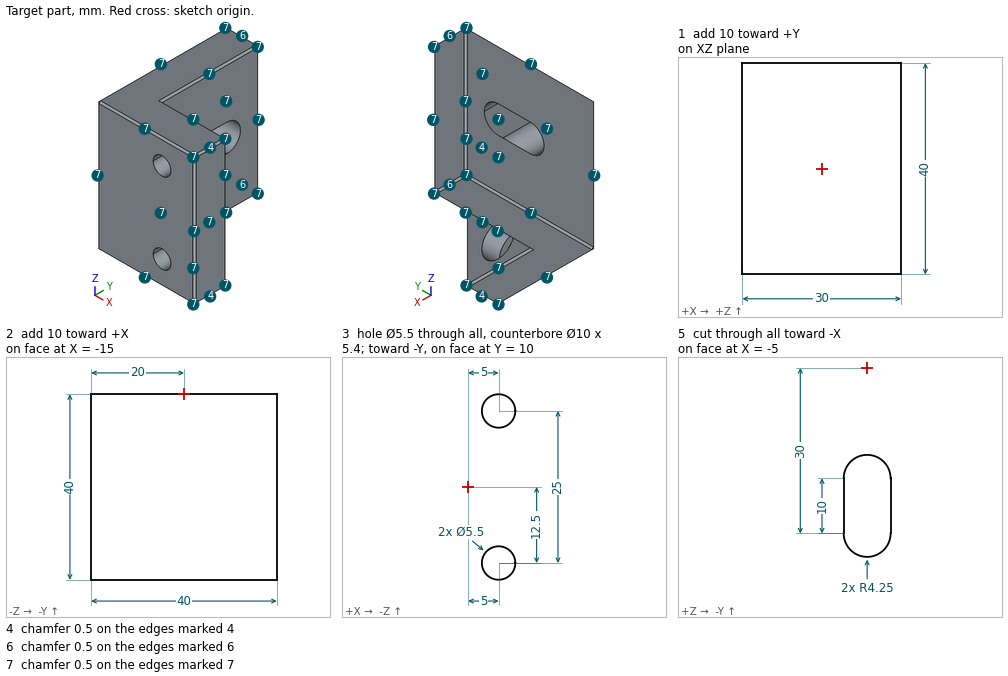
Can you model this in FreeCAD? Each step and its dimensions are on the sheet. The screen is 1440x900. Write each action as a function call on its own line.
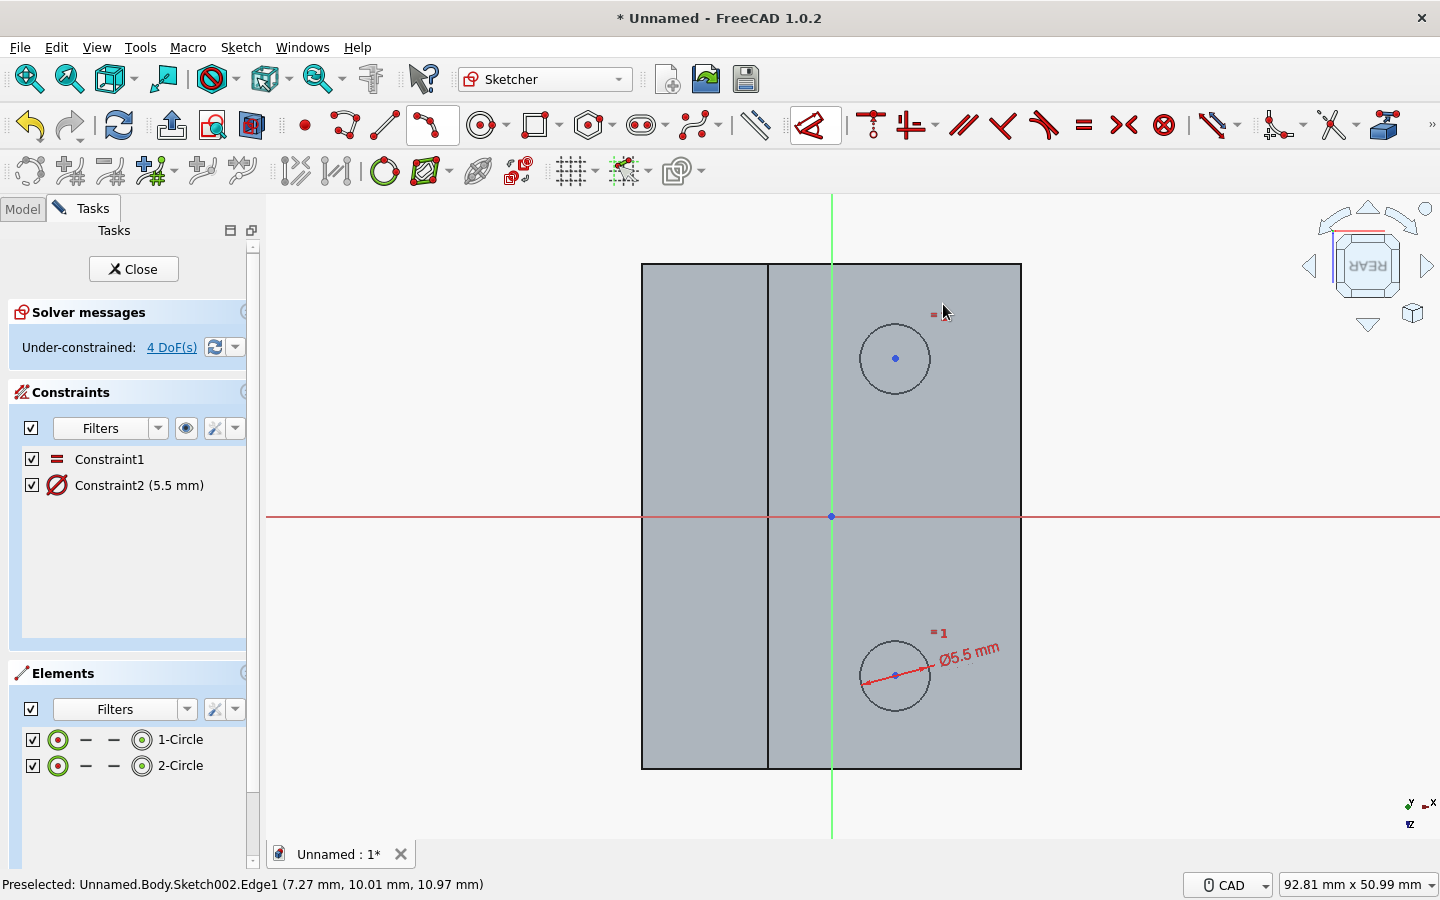
click(895, 676)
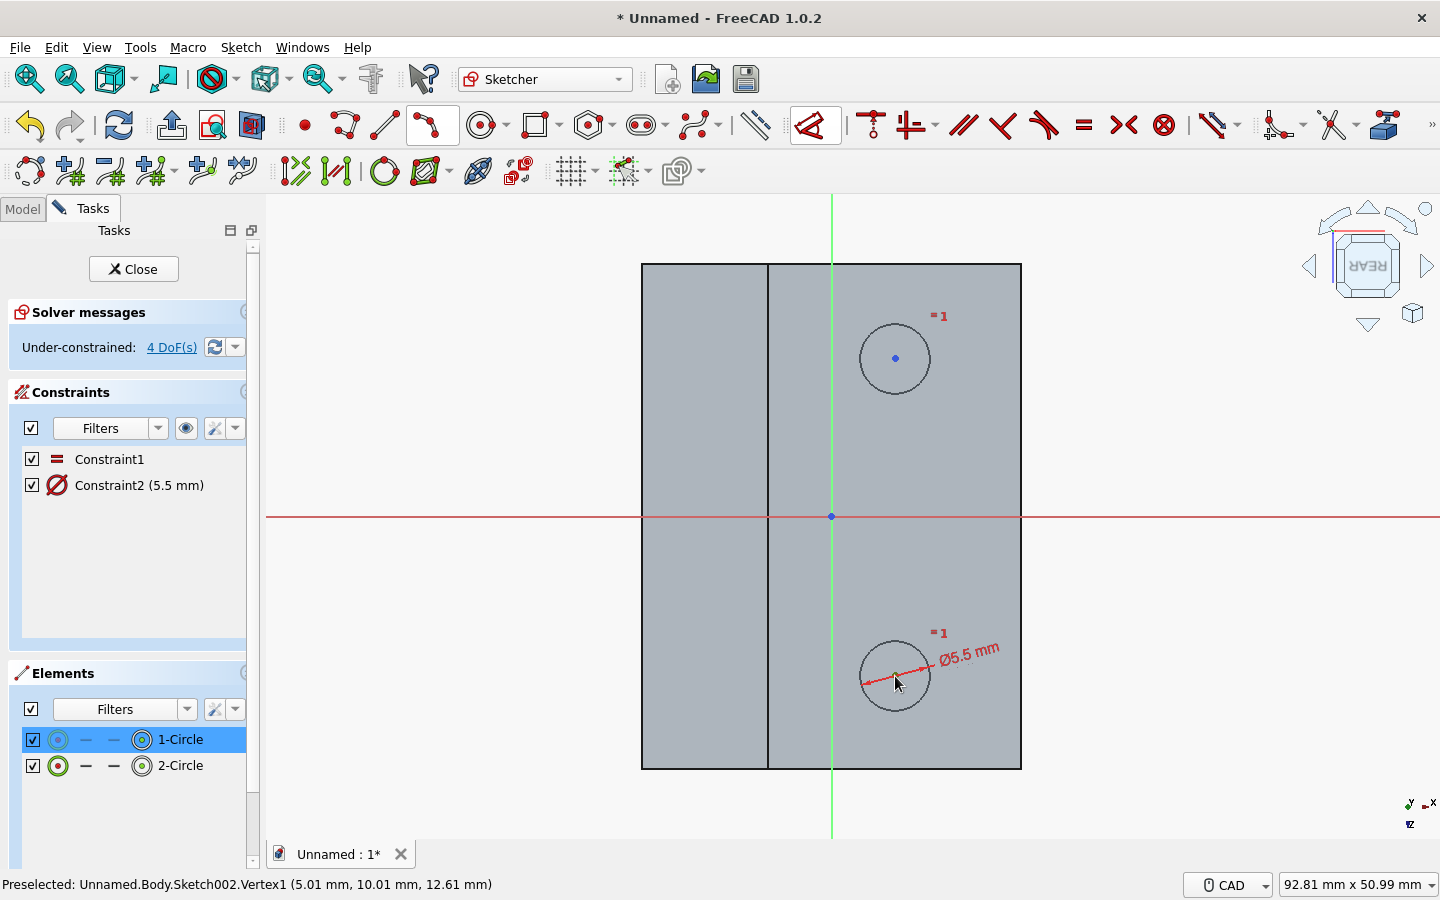
click(836, 126)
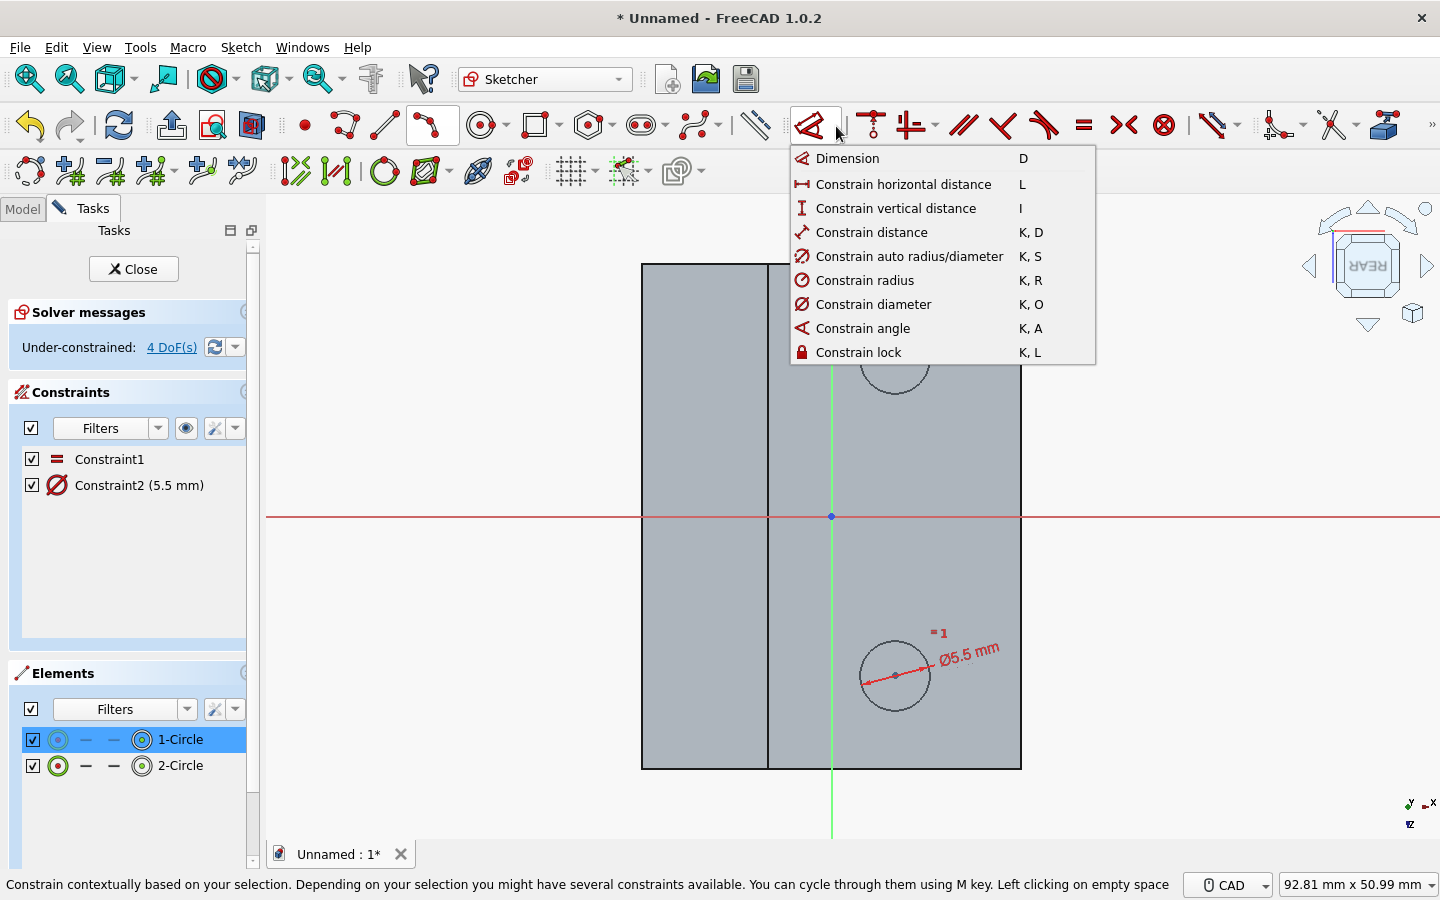
click(943, 184)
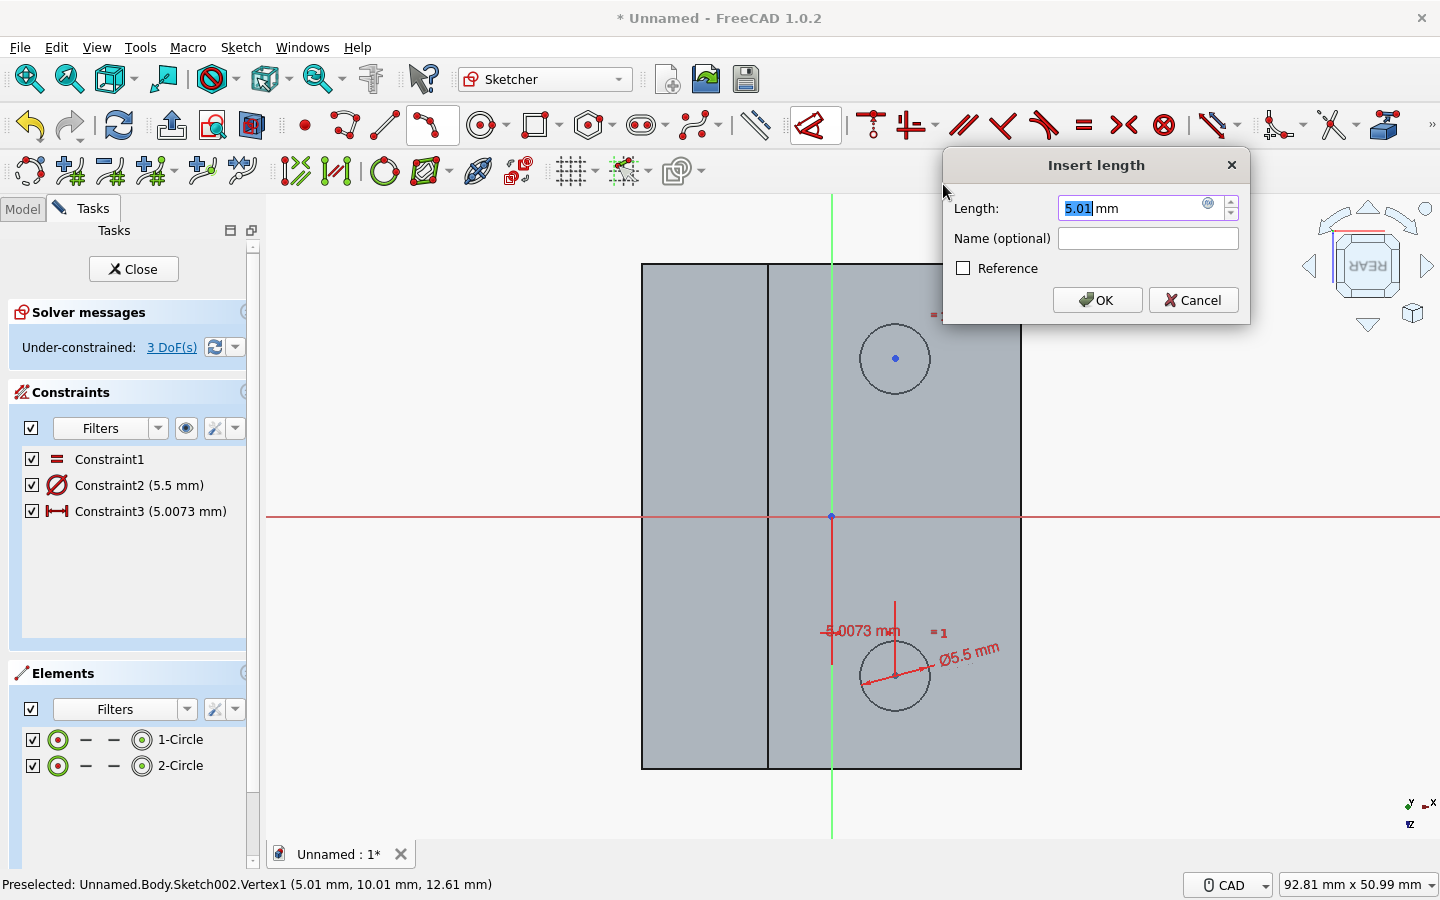
text(5)
key(Return)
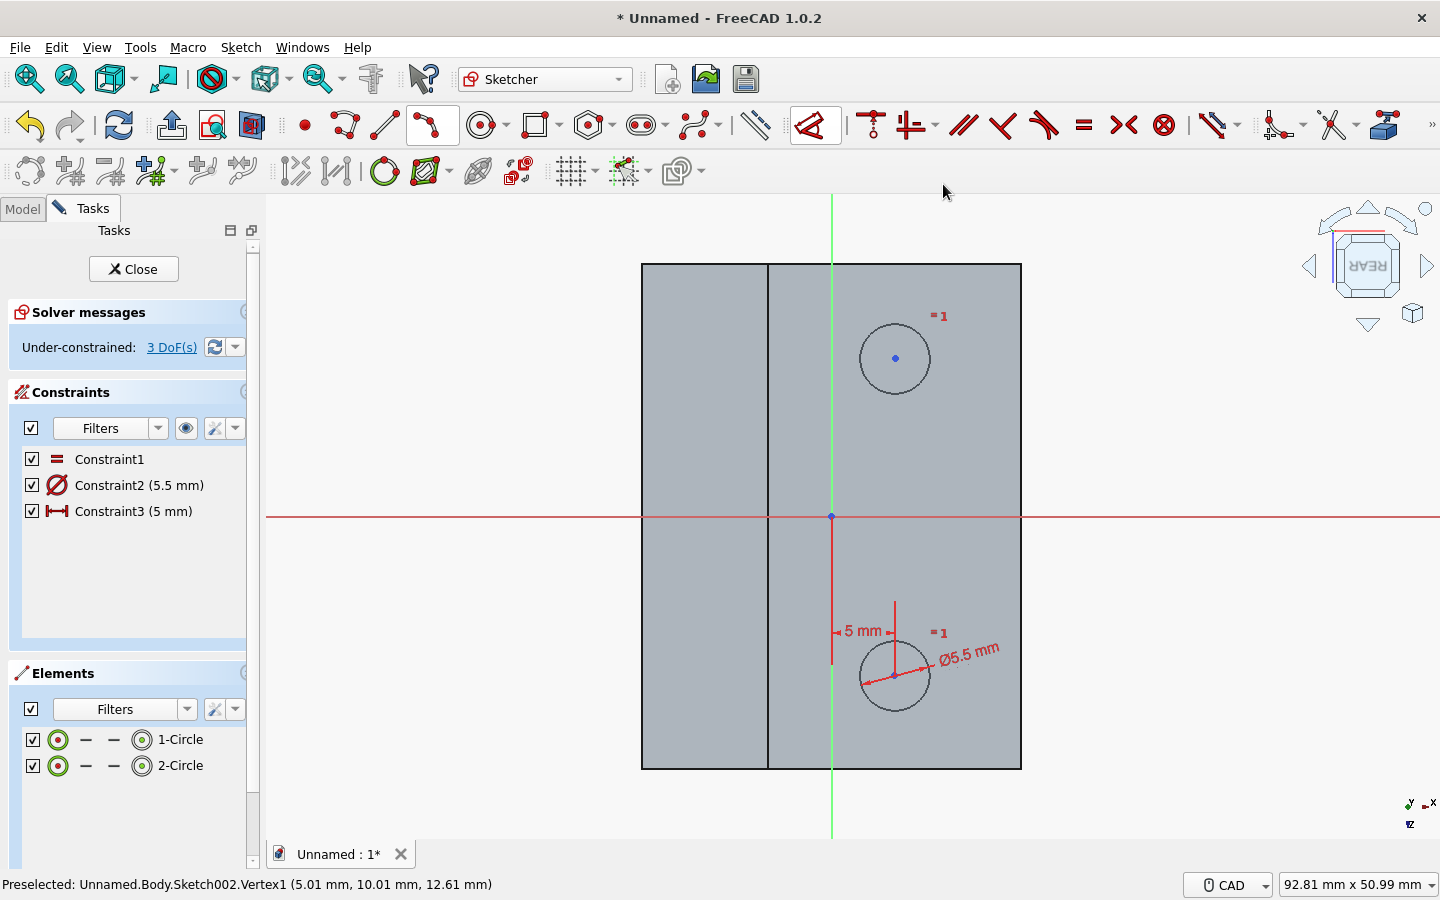
click(895, 359)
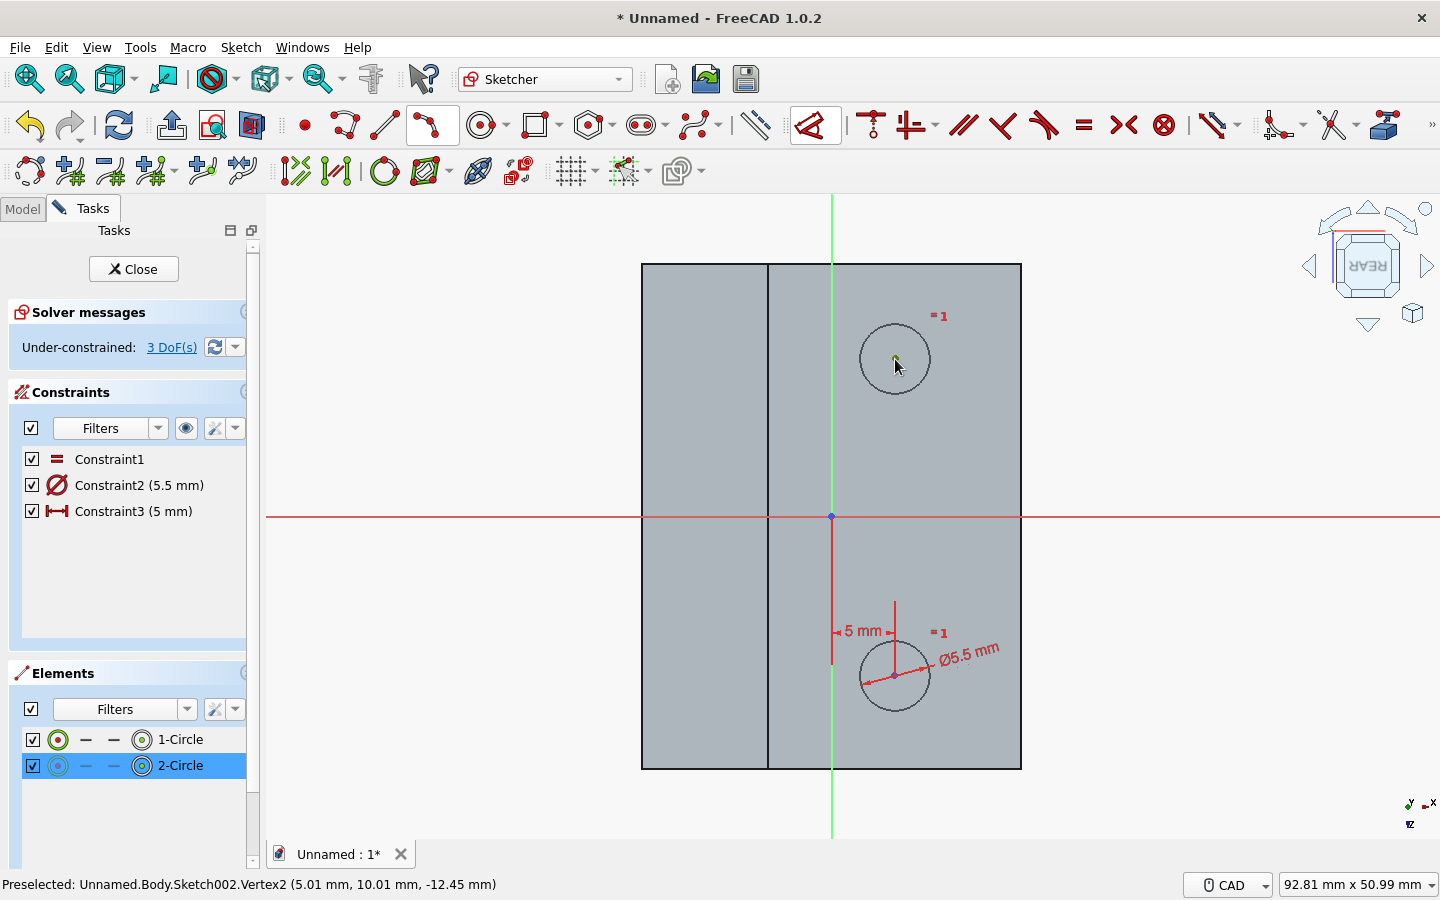
click(836, 126)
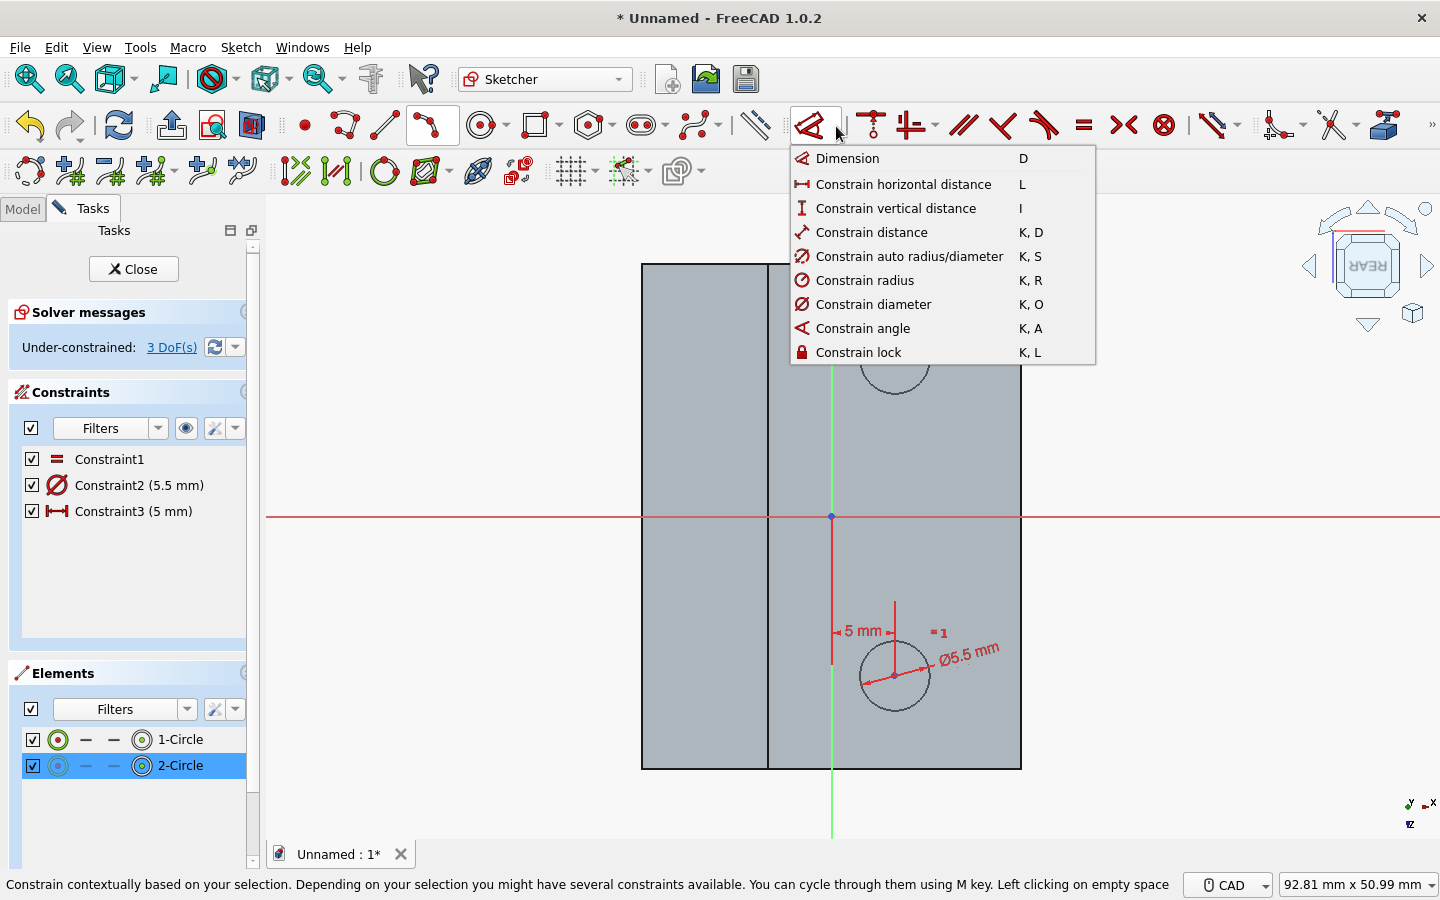
click(943, 184)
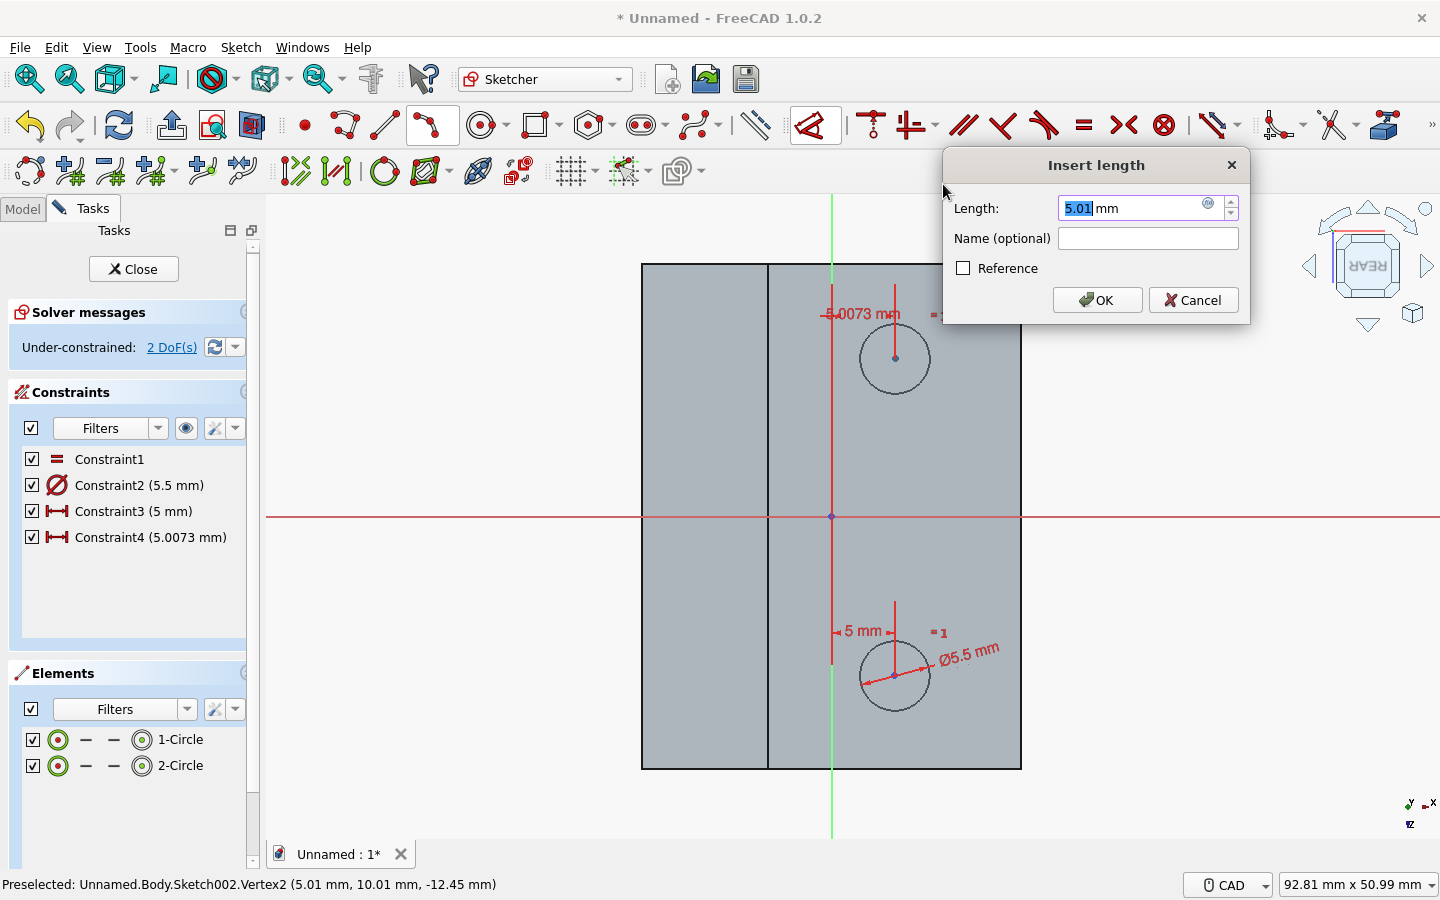
text(5)
key(Return)